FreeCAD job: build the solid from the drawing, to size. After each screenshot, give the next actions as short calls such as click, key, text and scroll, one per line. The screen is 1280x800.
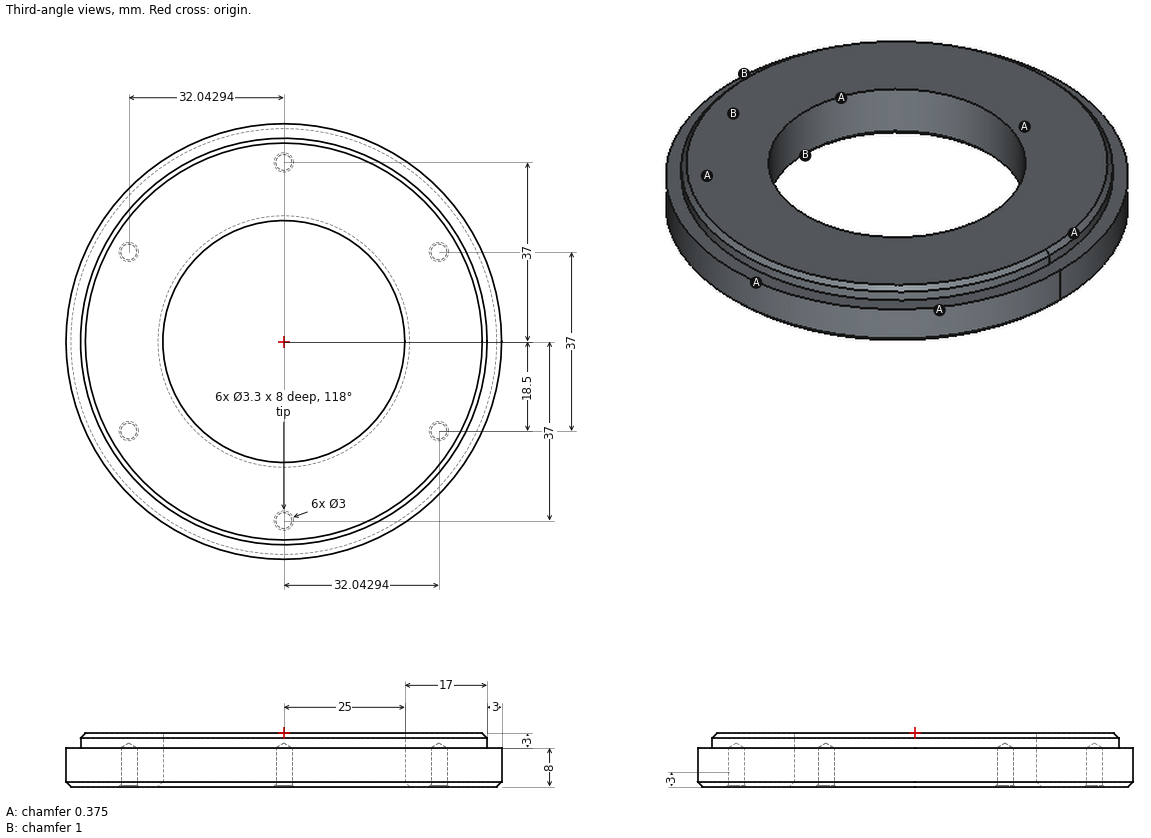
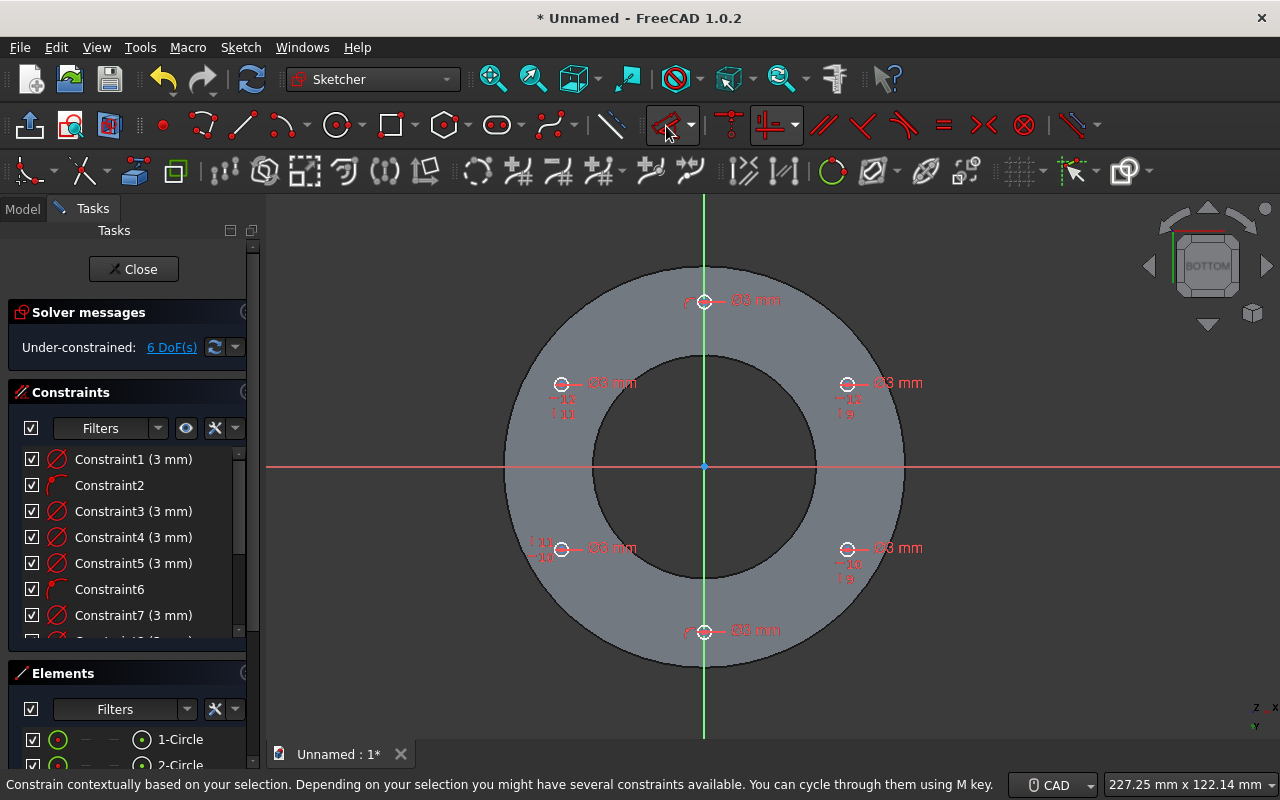
click(704, 302)
click(738, 385)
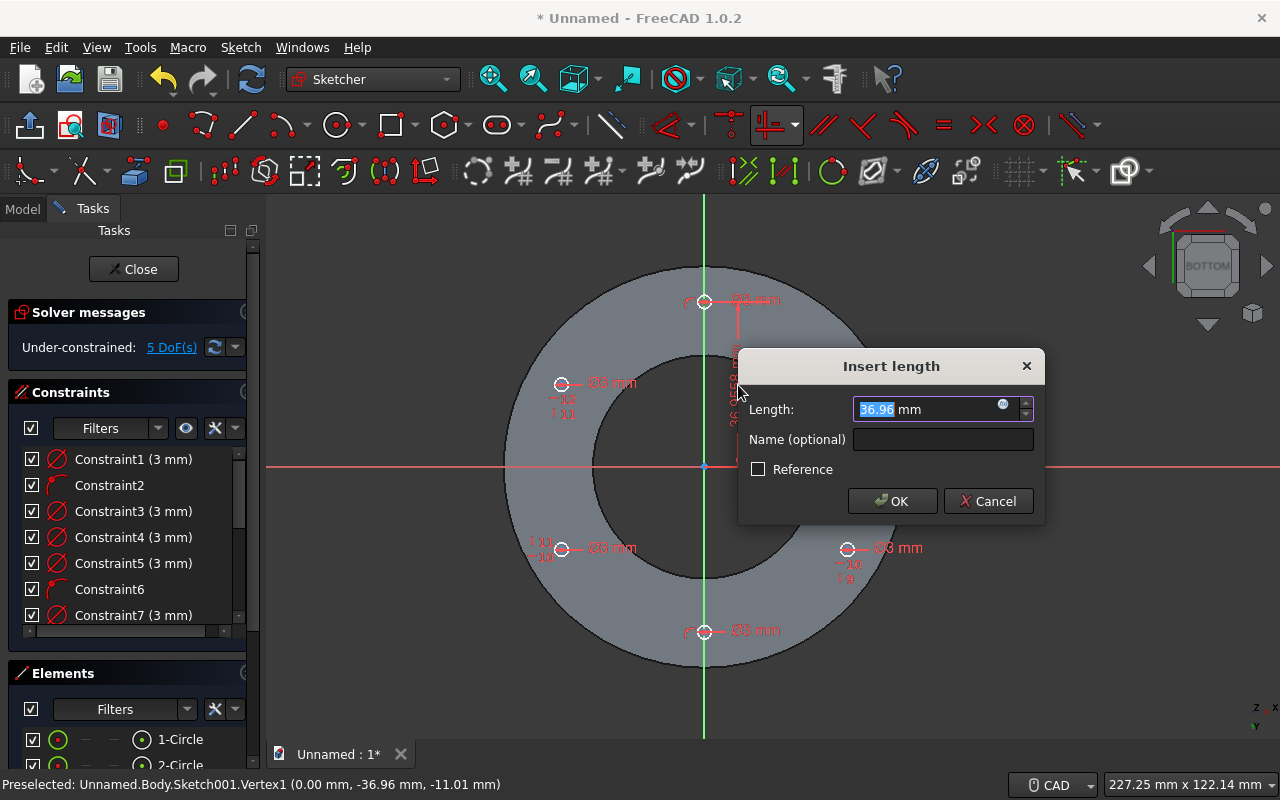
text(37)
key(Return)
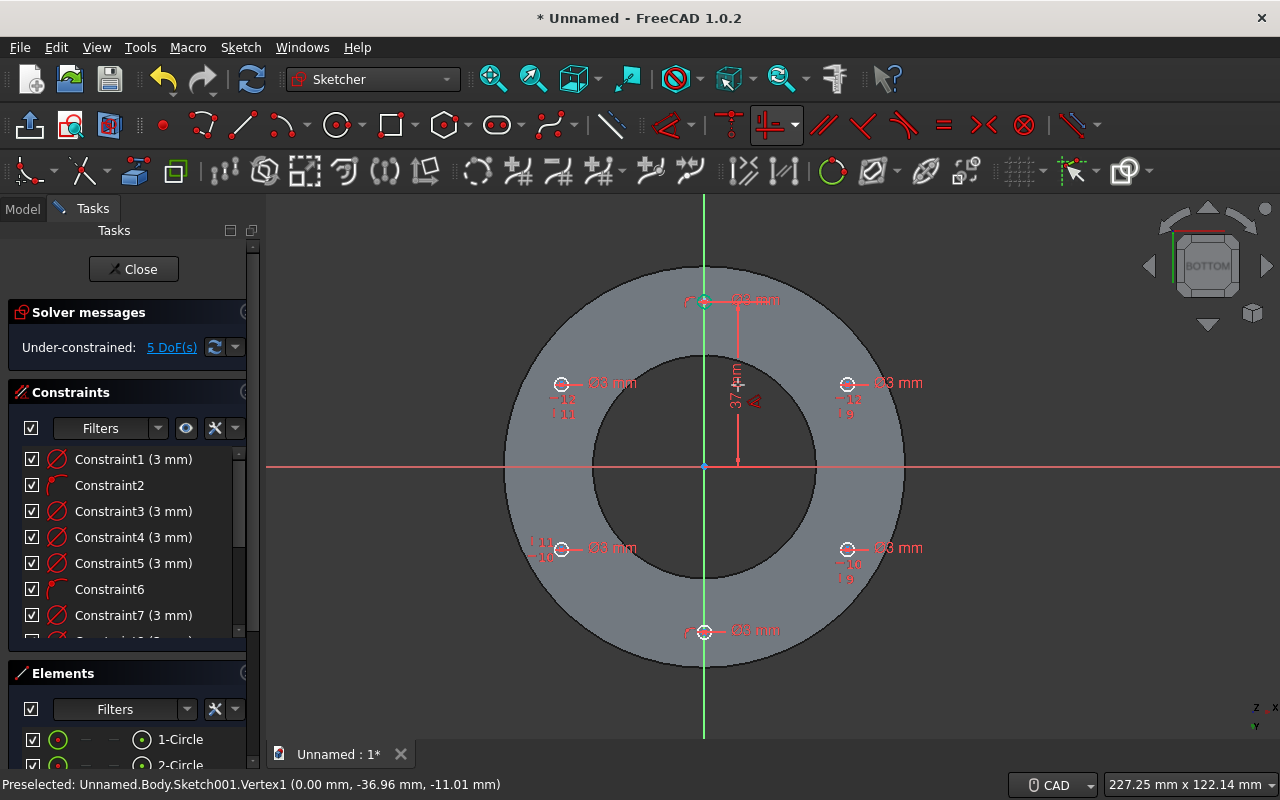
click(704, 632)
click(738, 550)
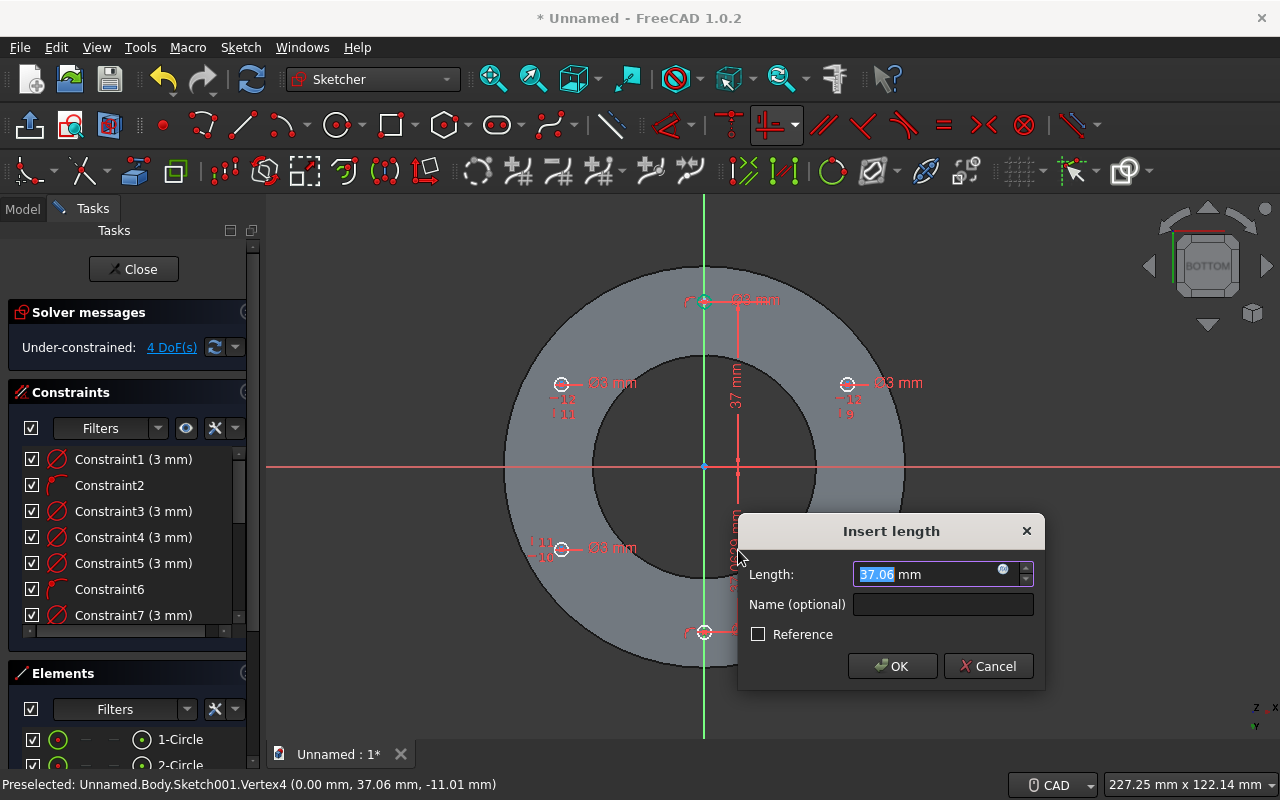
text(37)
key(Return)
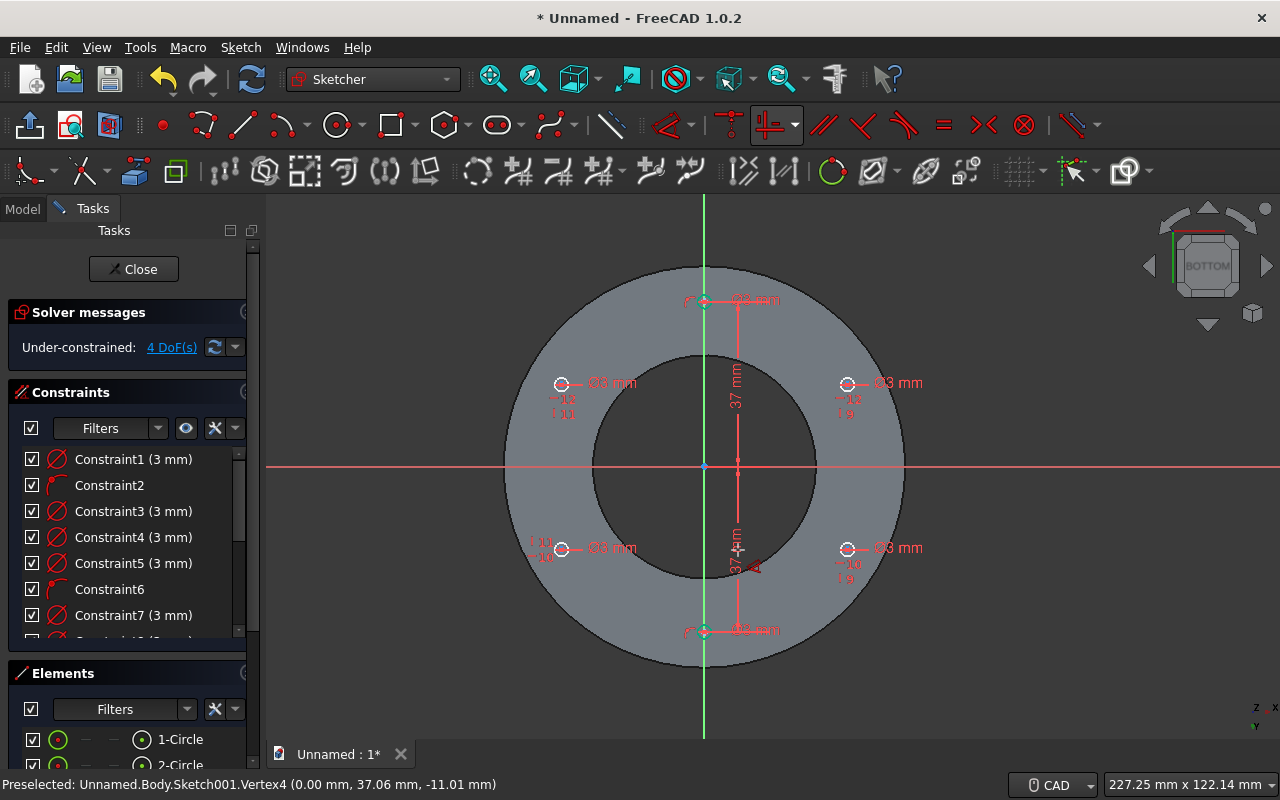
click(847, 385)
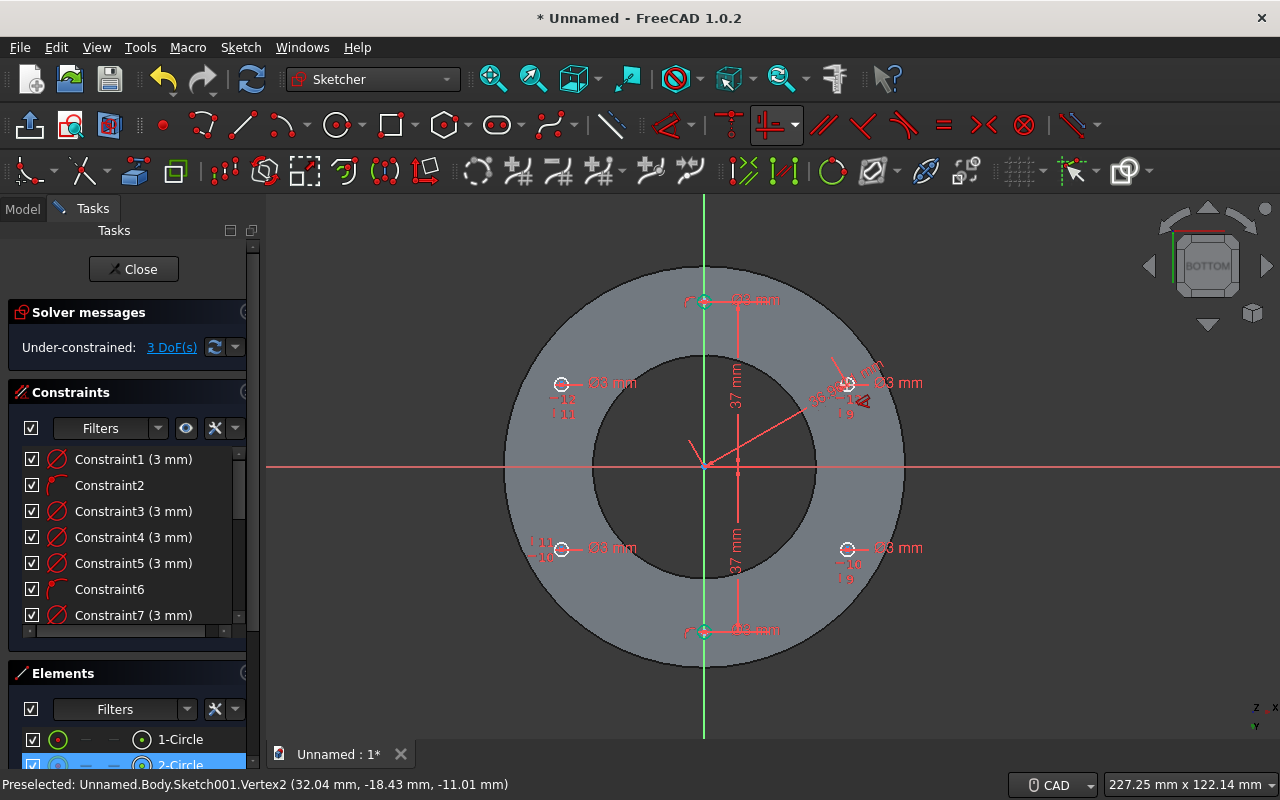
click(847, 550)
click(881, 429)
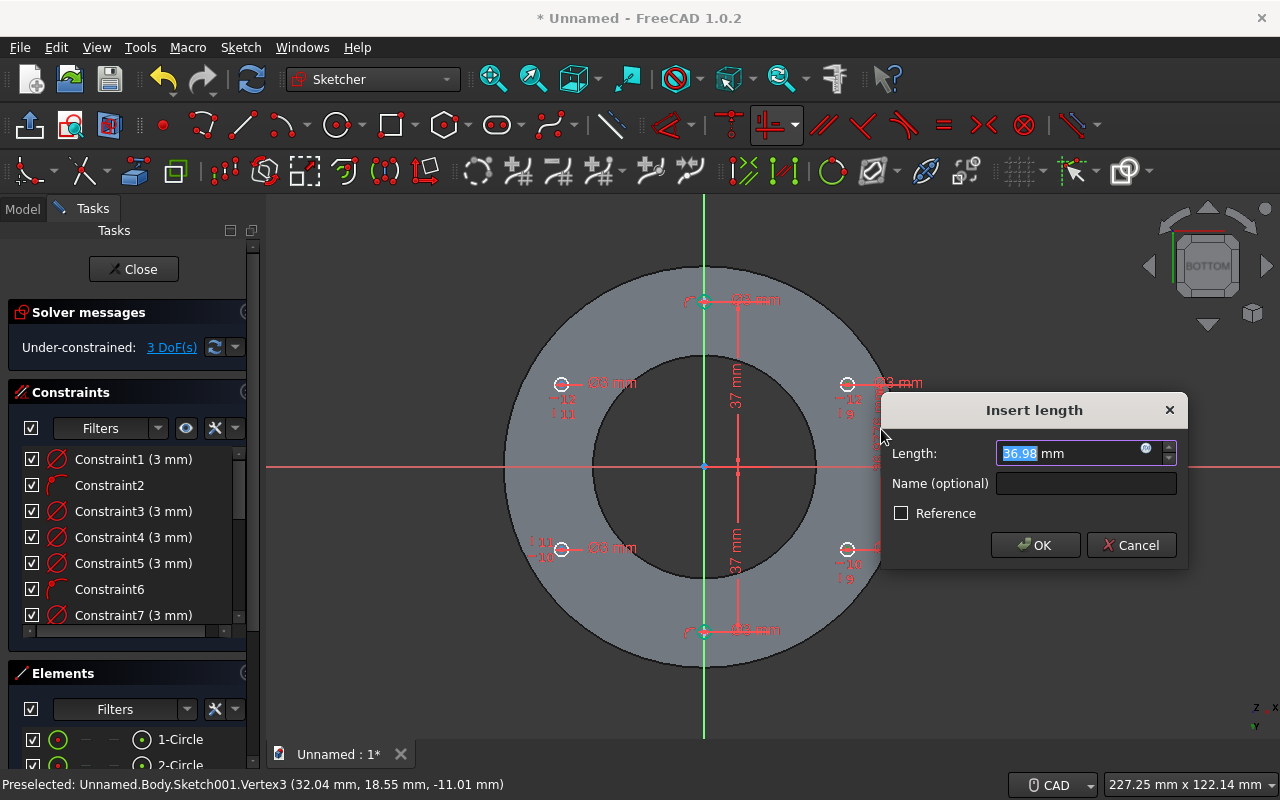
text(37)
key(Return)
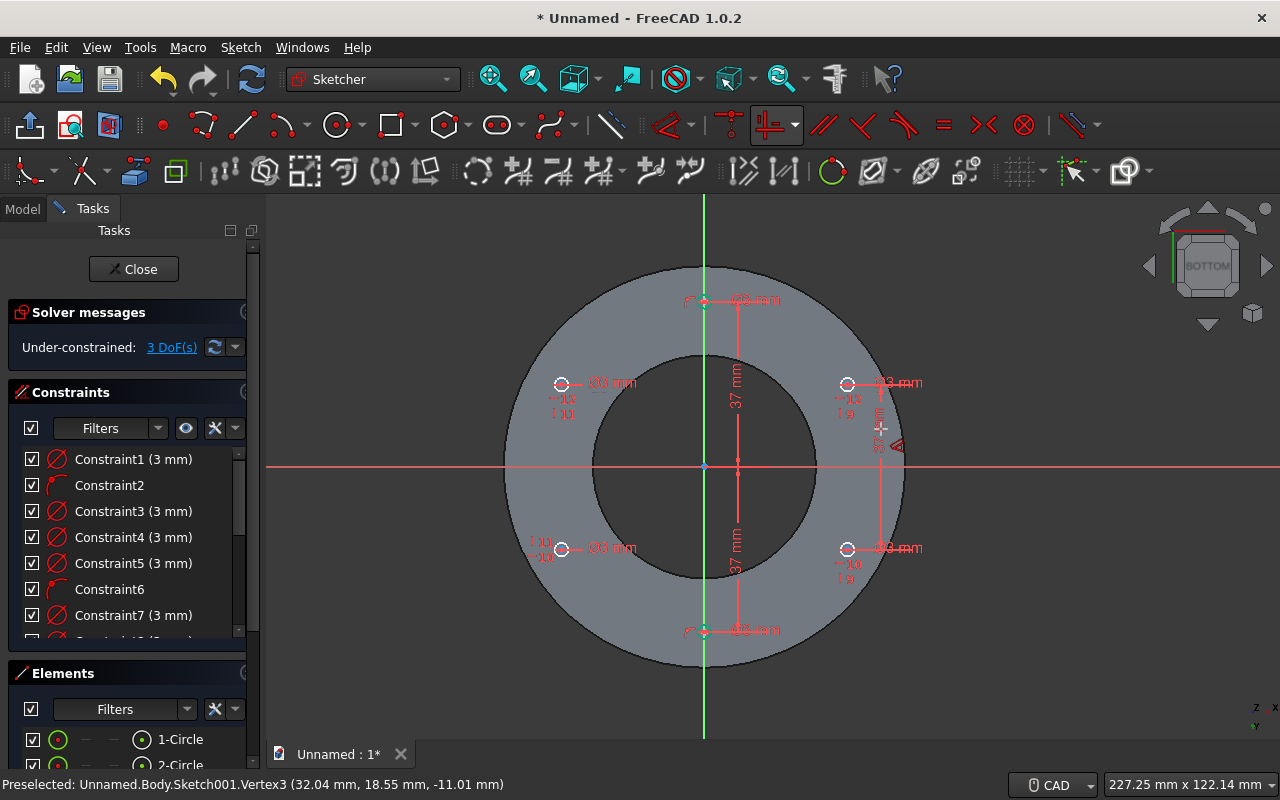
click(847, 385)
click(881, 407)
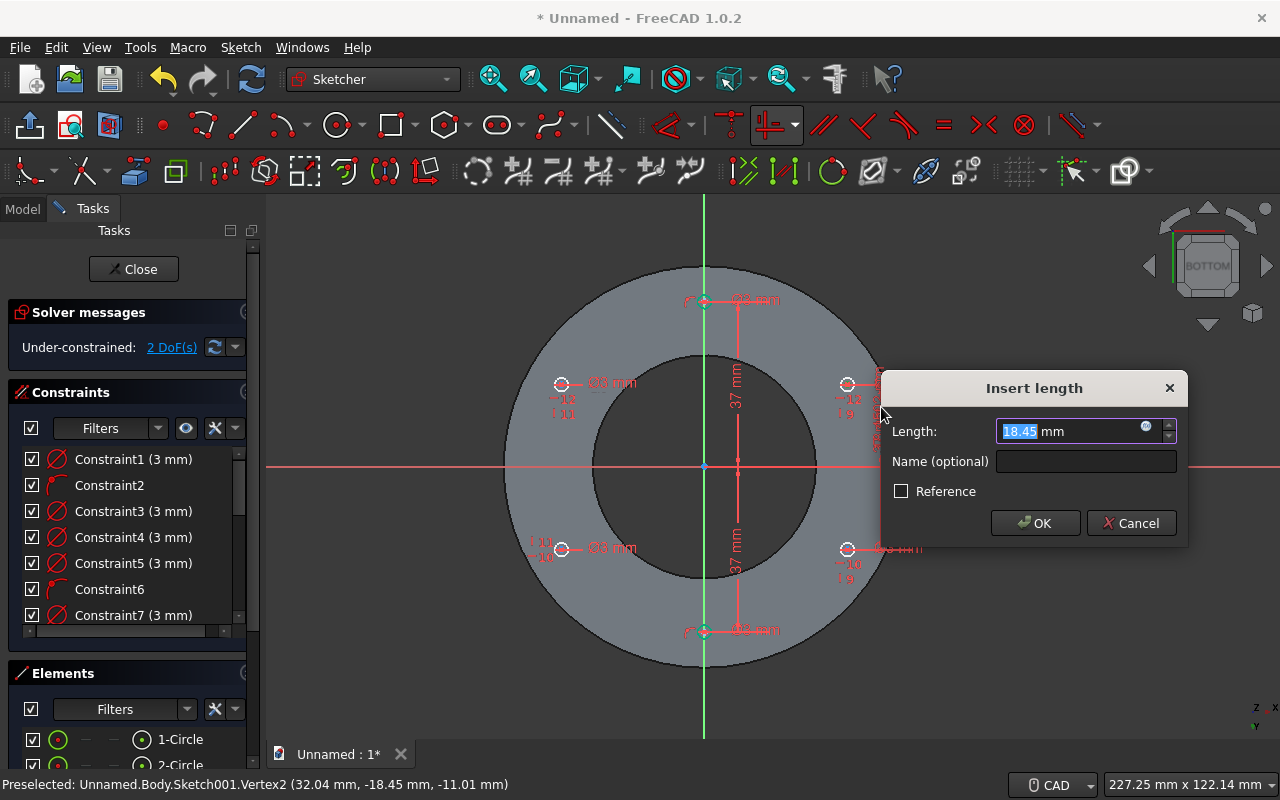
text(18.5)
key(Return)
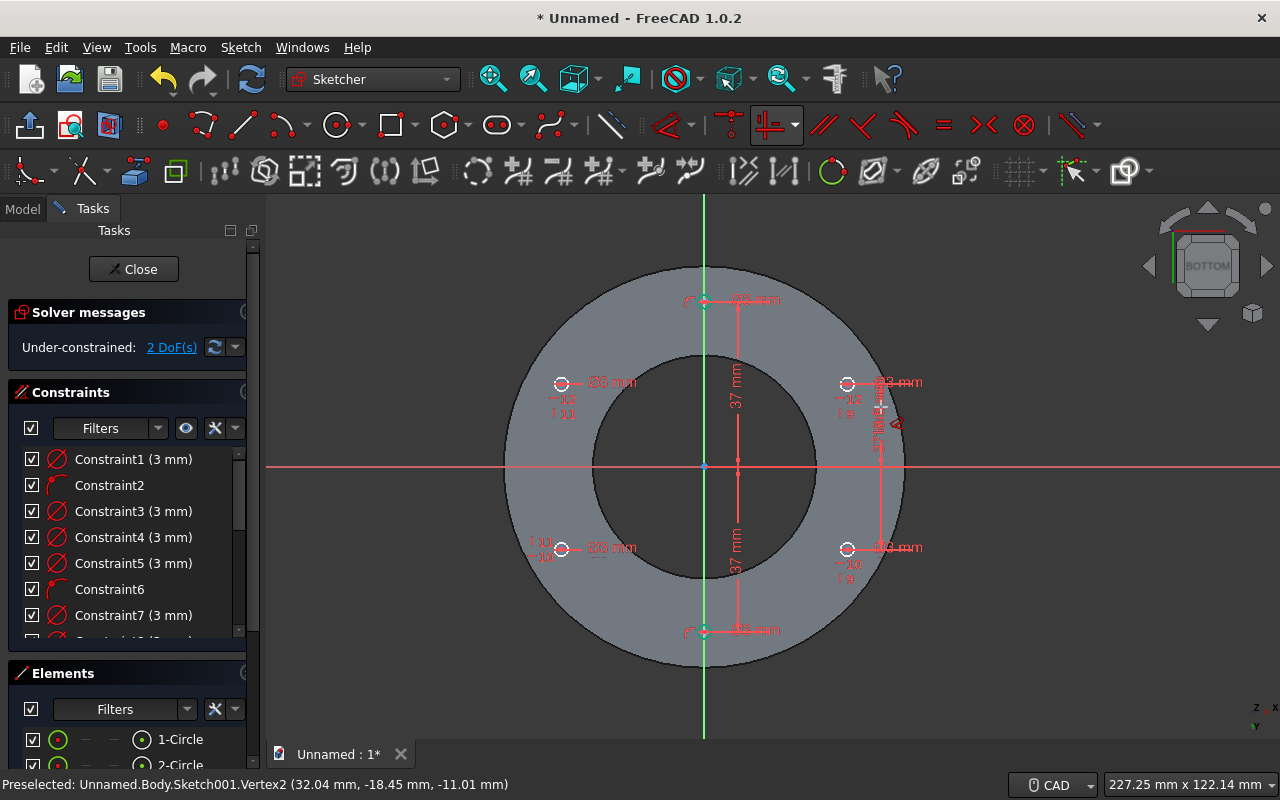
click(847, 384)
click(776, 350)